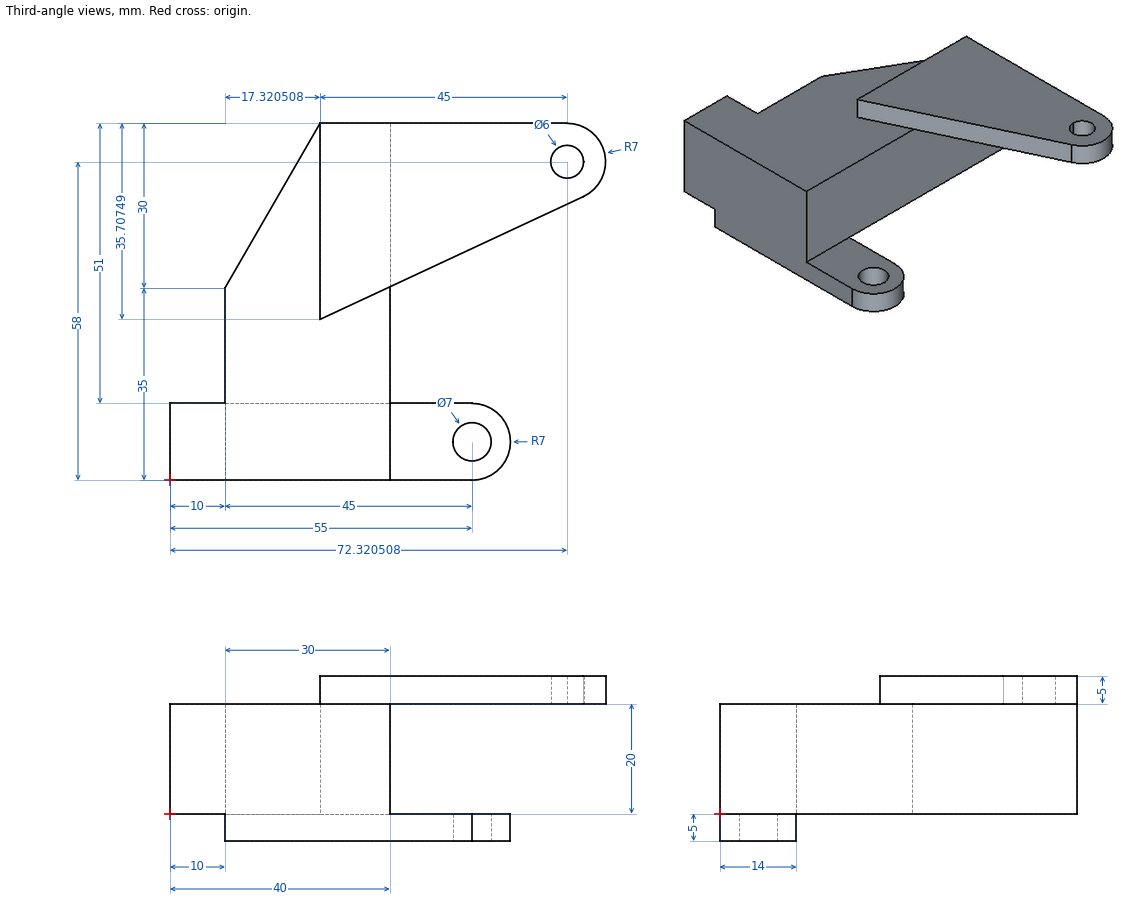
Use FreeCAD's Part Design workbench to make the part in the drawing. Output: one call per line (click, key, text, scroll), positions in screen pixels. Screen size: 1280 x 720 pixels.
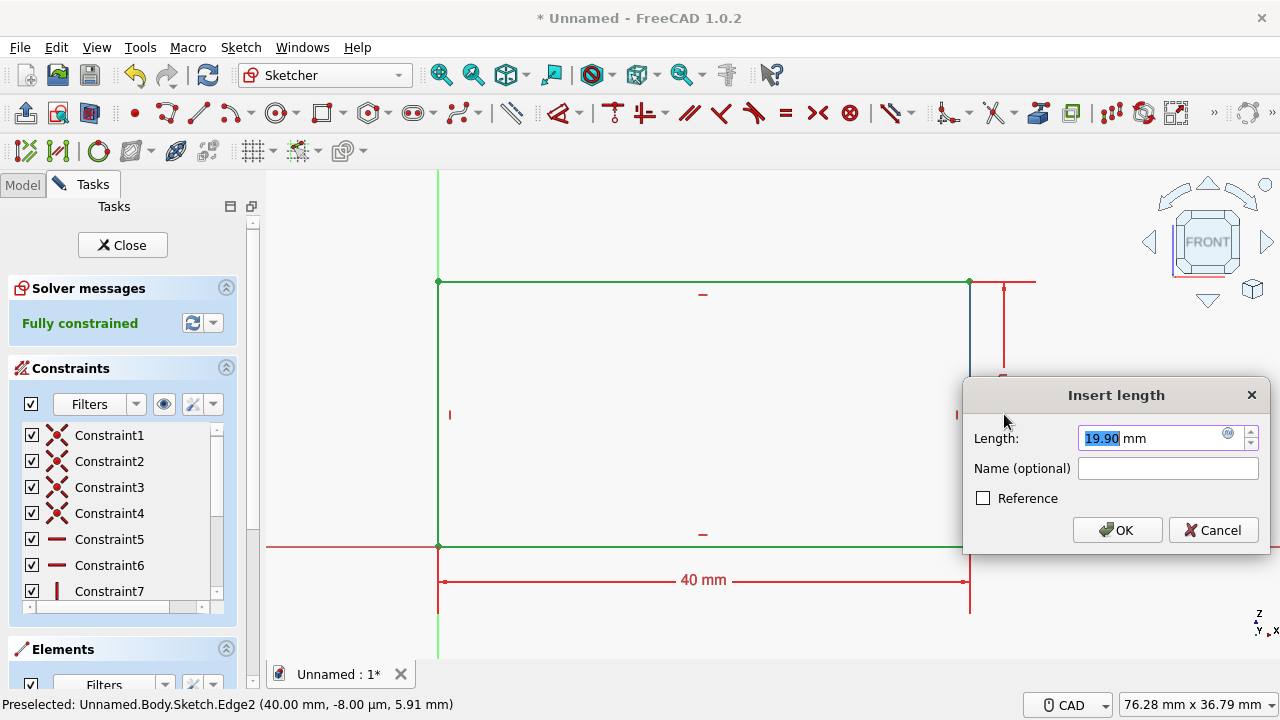
text(20)
key(Return)
key(Escape)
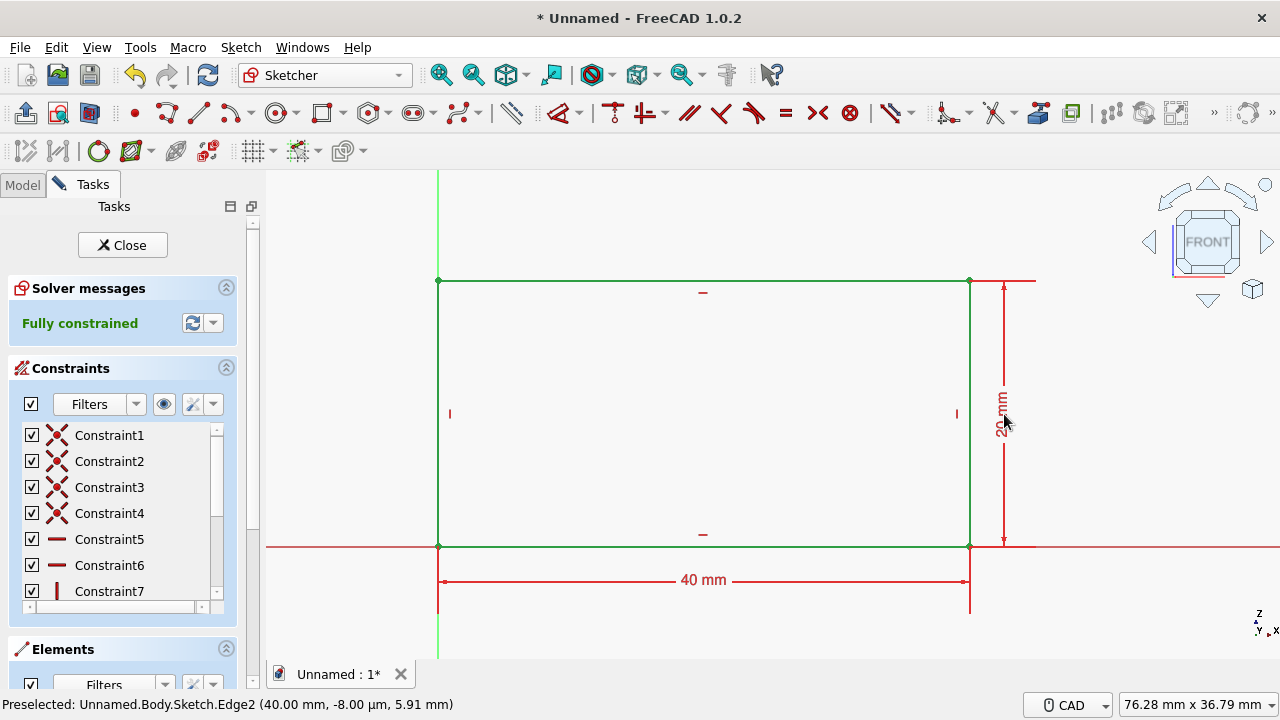
click(123, 245)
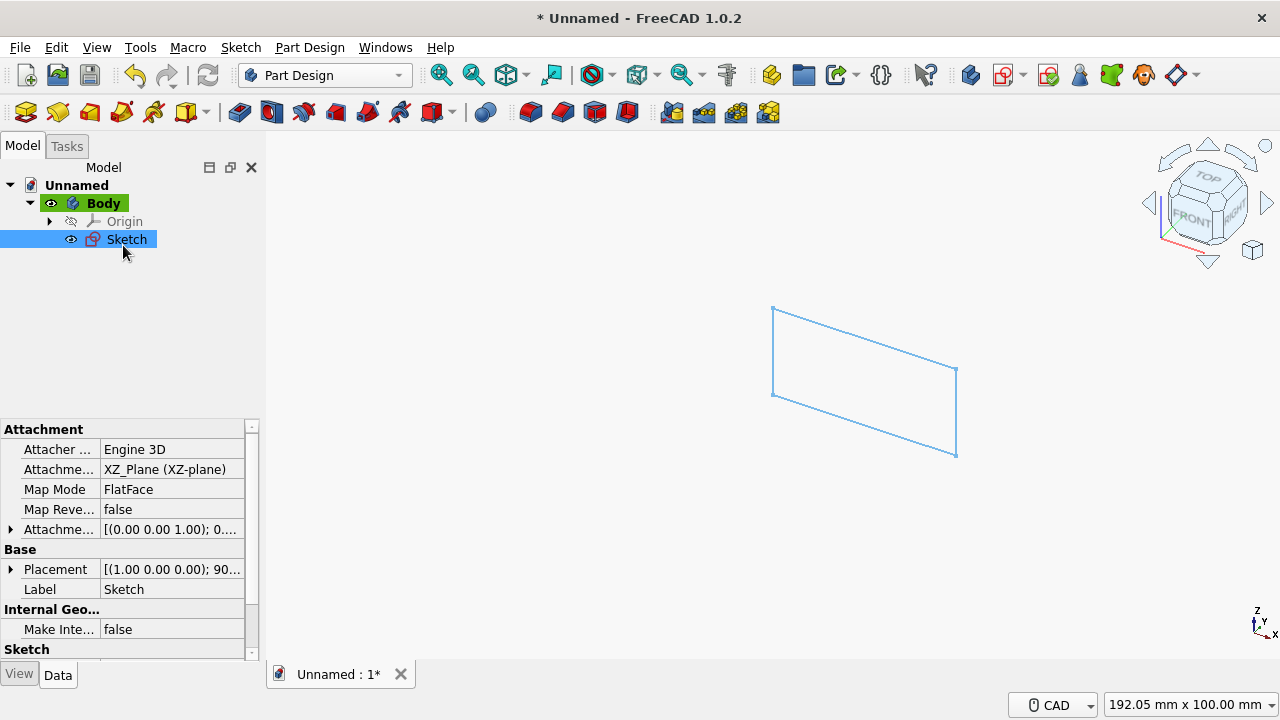
click(26, 112)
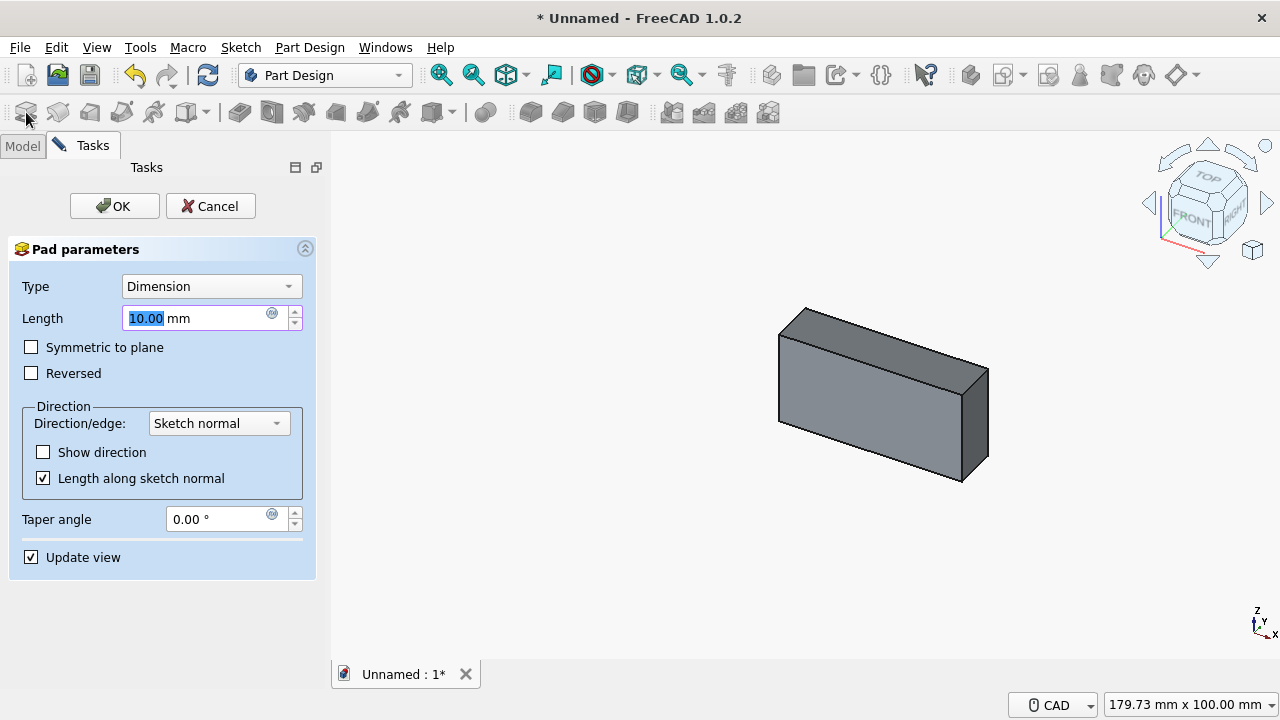
text(14)
key(Tab)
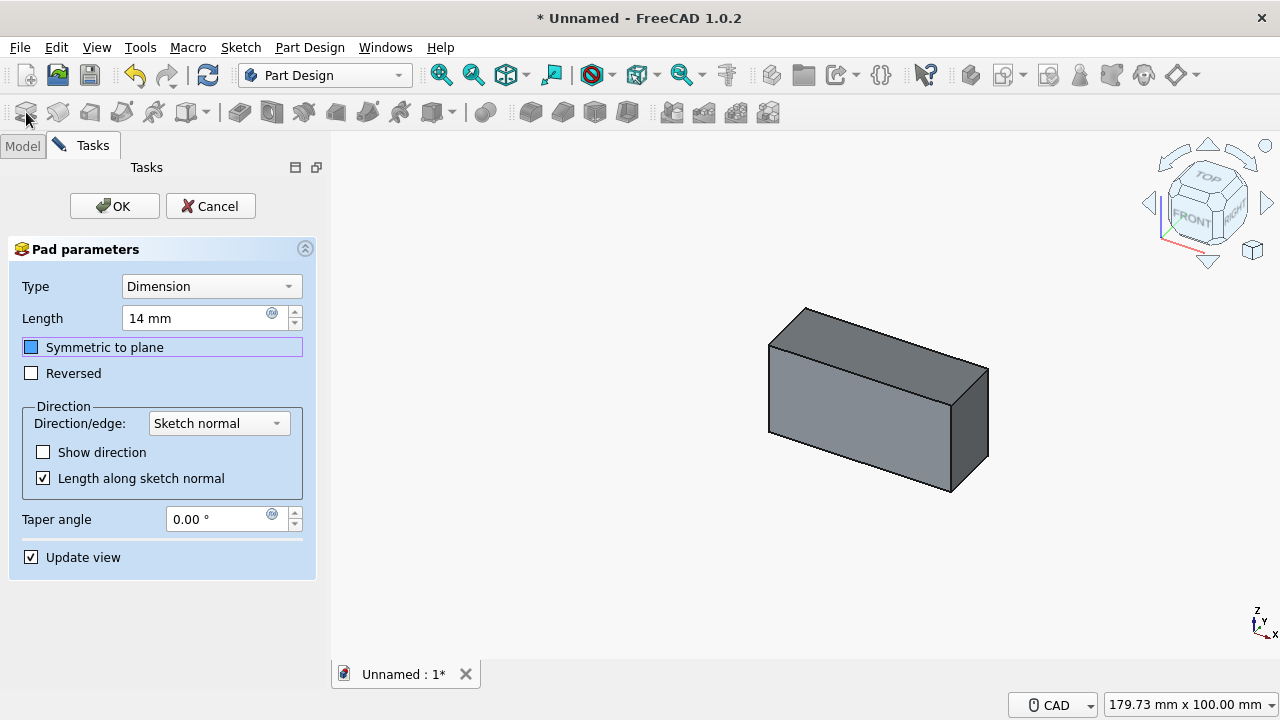
click(30, 373)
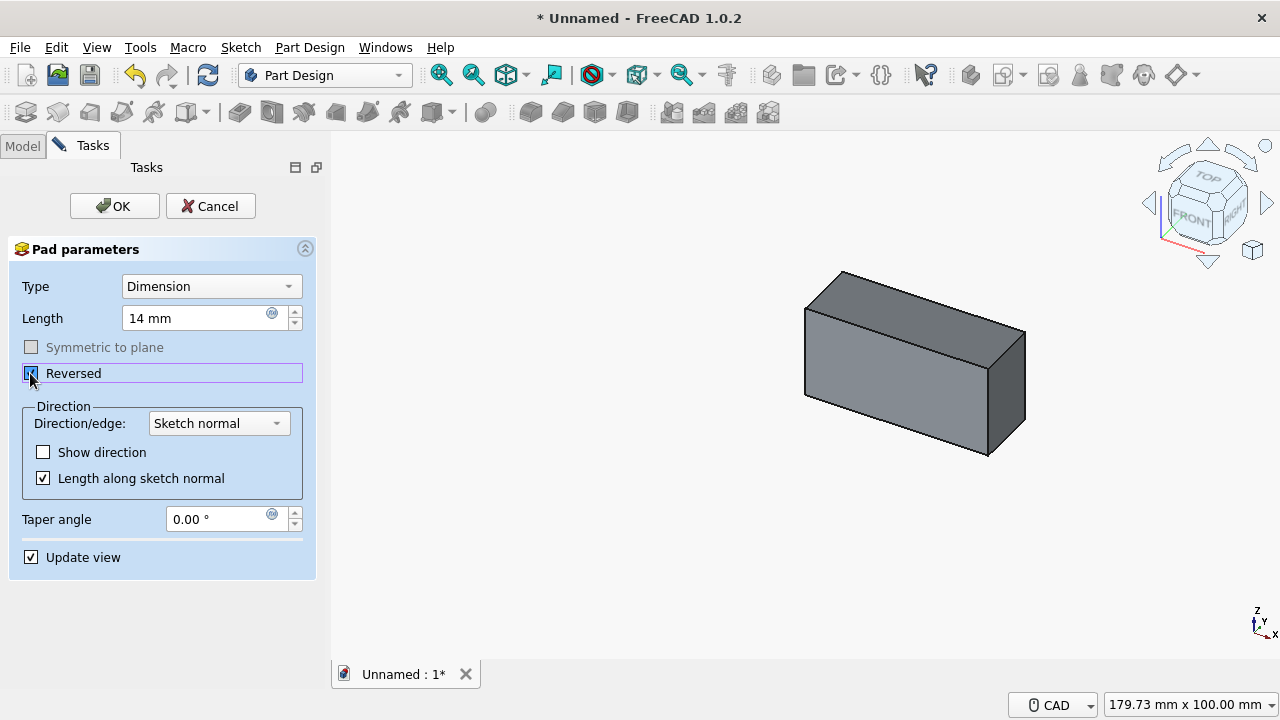
click(115, 206)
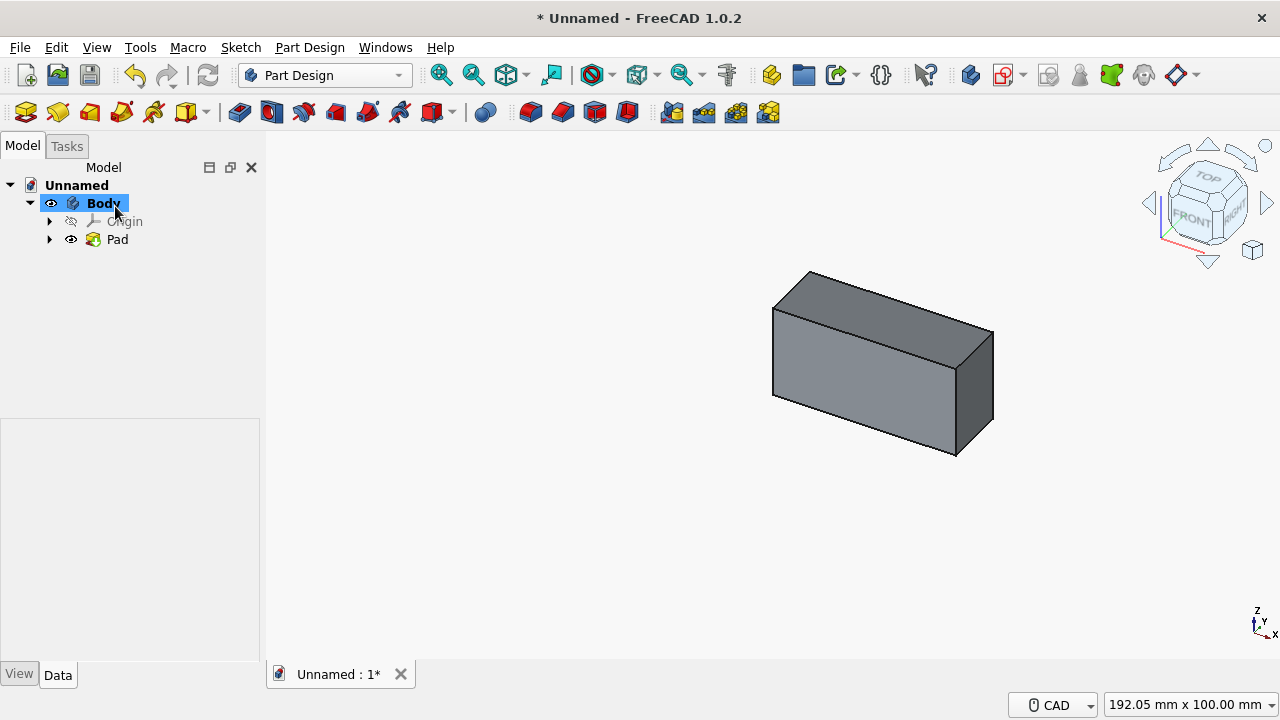
click(442, 76)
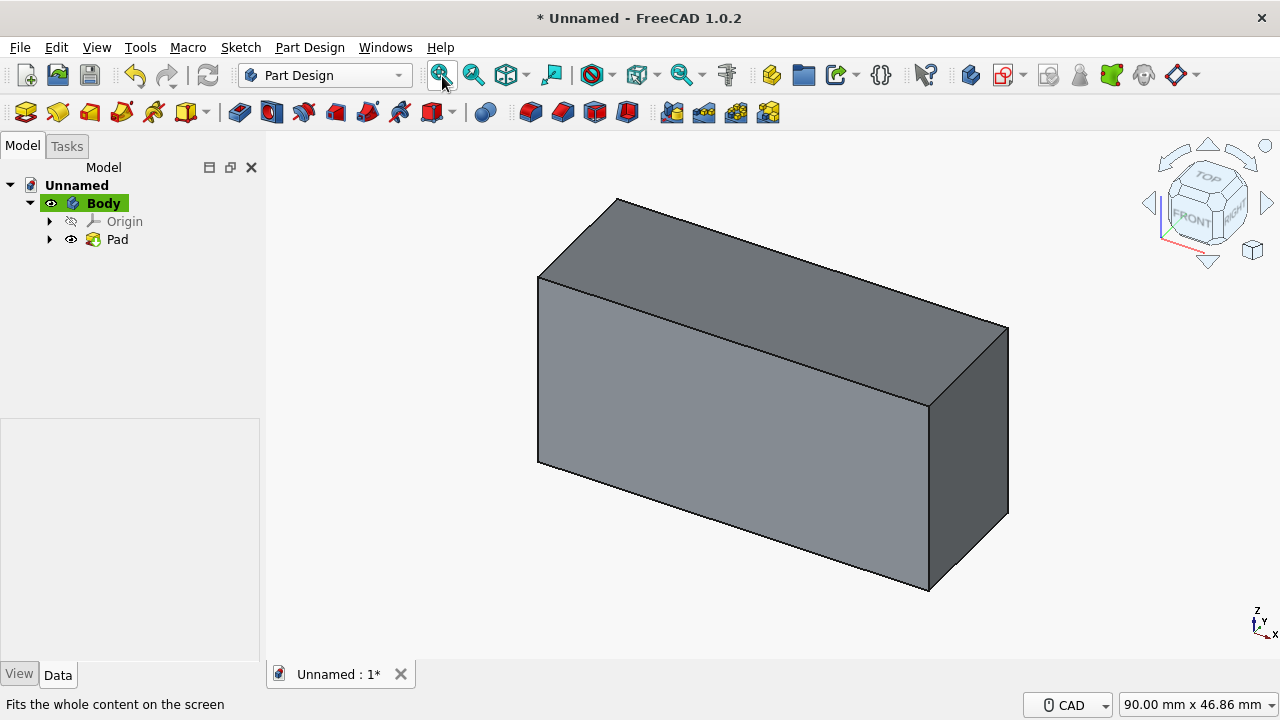
key(4)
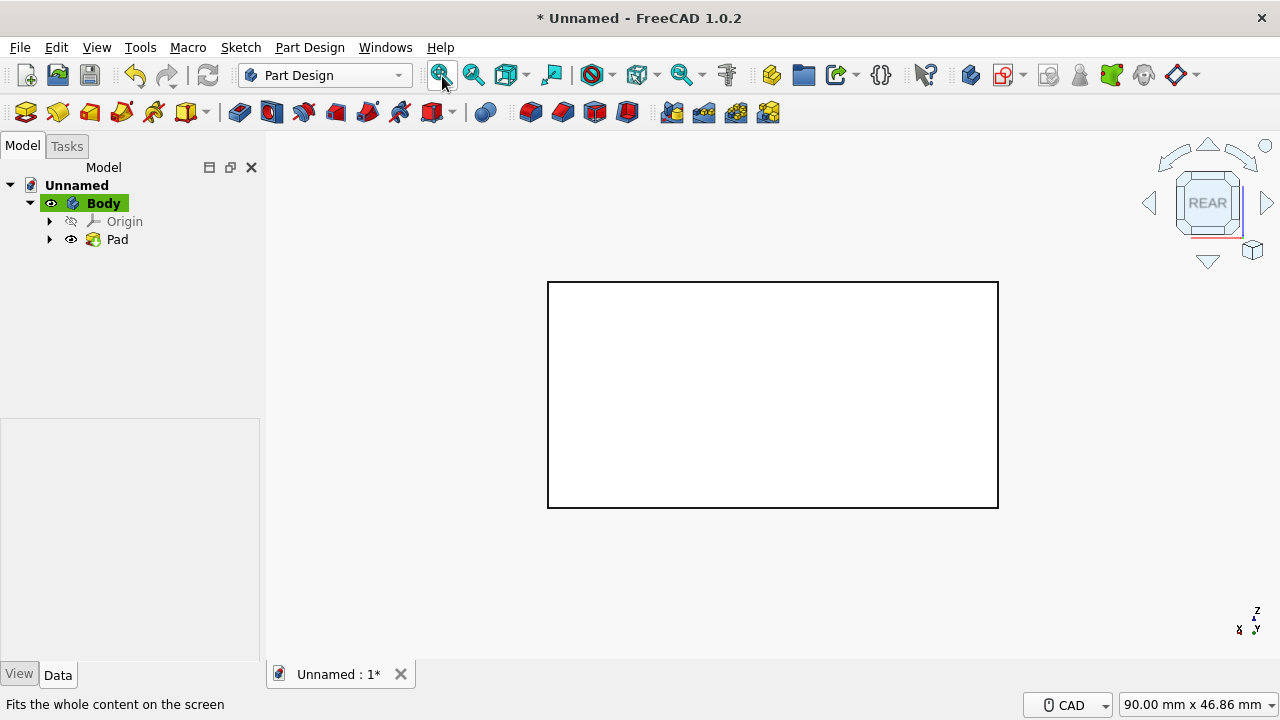
click(442, 76)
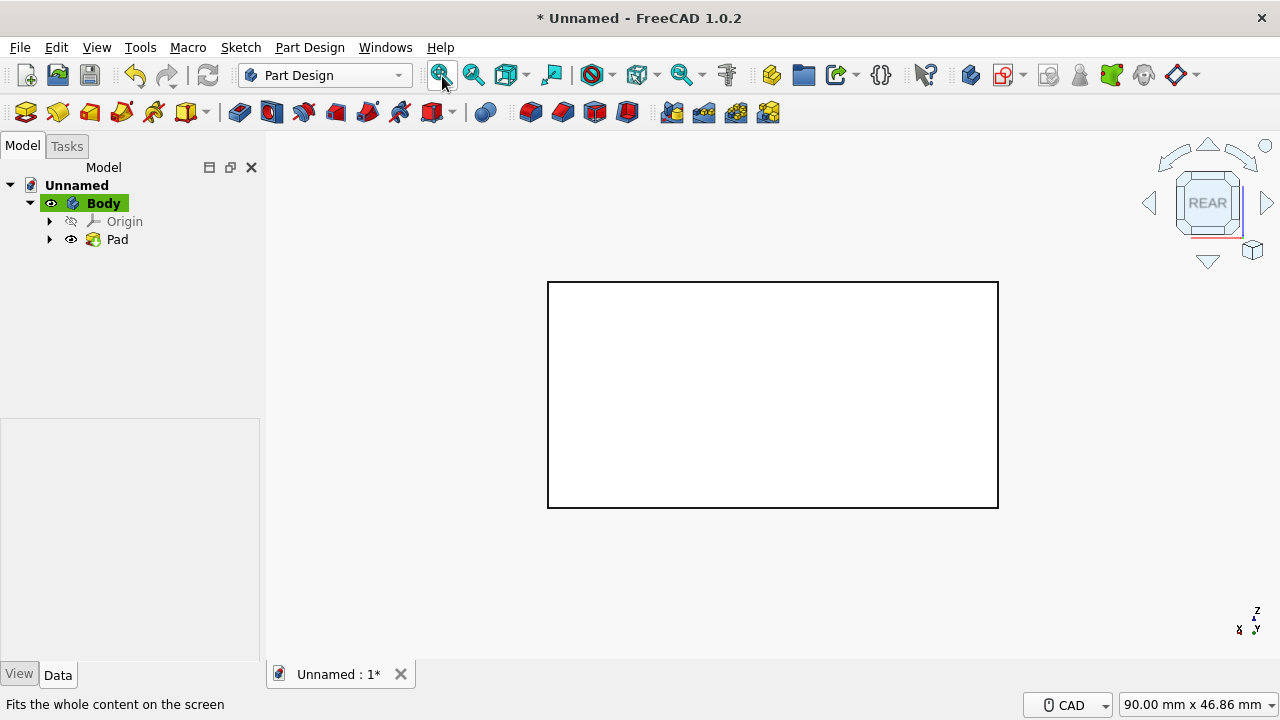
click(709, 394)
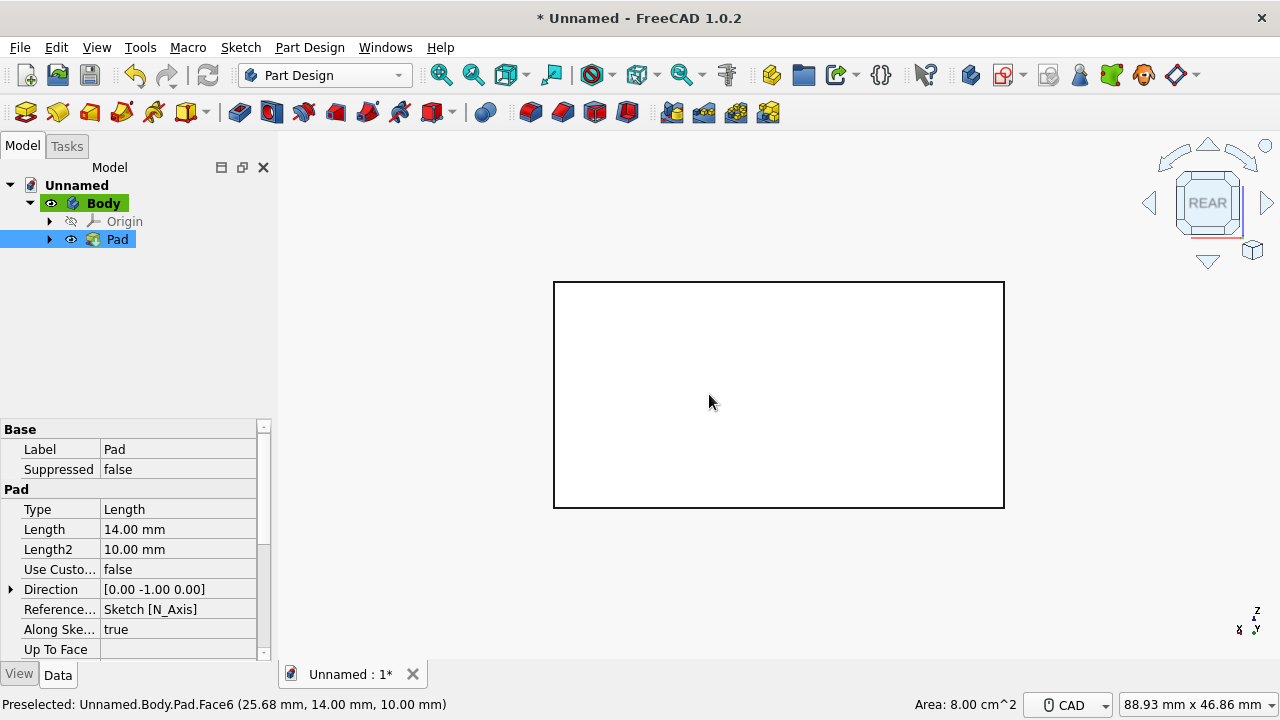
click(1004, 76)